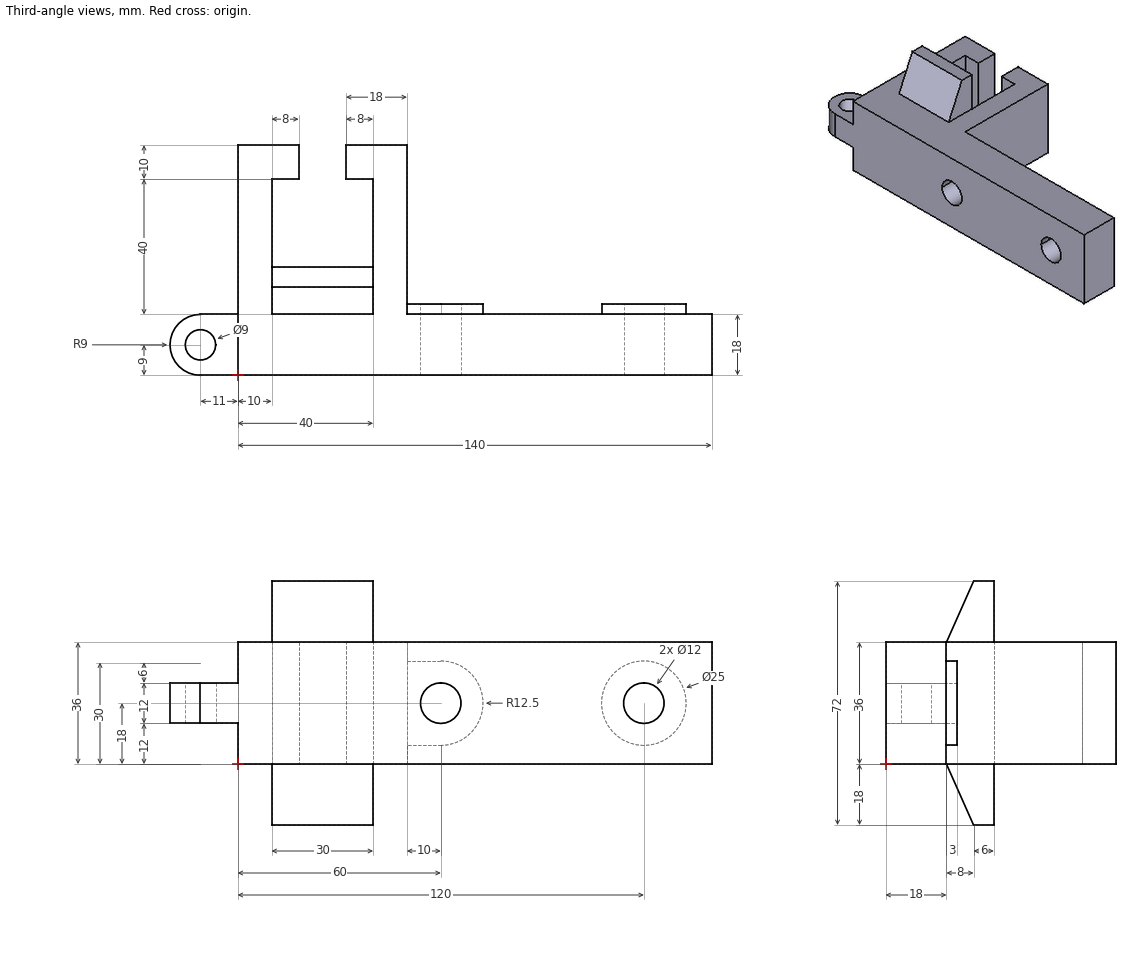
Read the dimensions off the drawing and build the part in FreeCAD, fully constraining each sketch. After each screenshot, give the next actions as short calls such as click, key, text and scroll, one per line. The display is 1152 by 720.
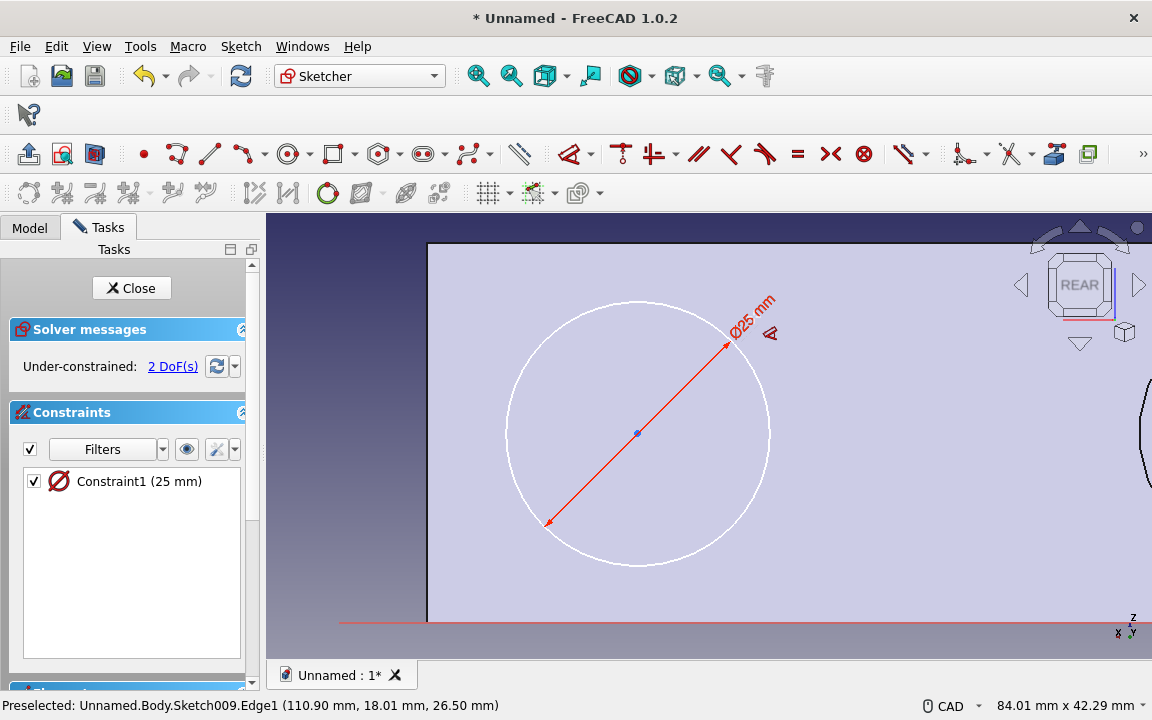
click(638, 434)
click(604, 528)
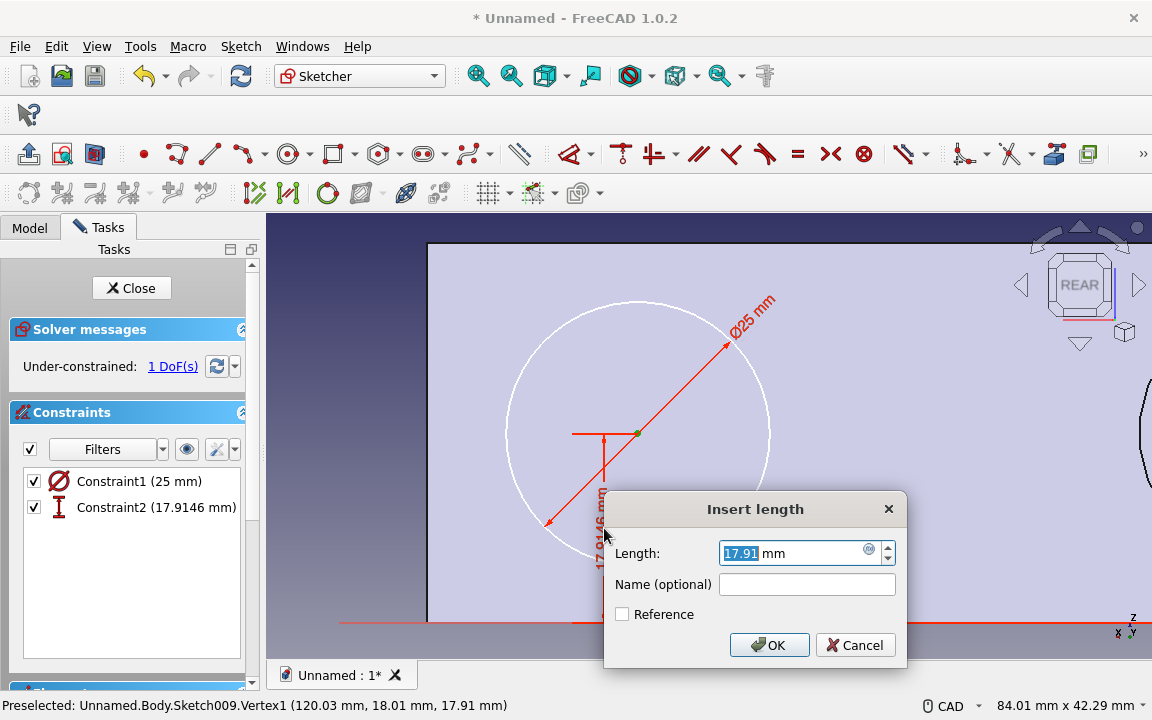
text(18)
key(Return)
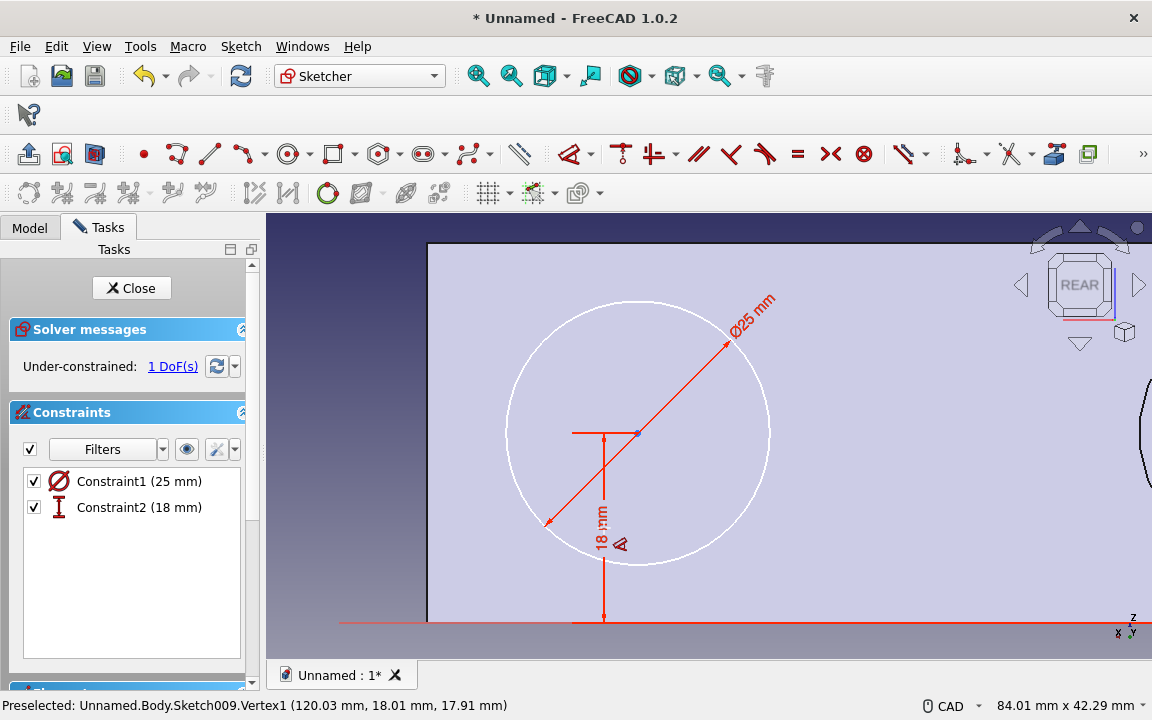
click(638, 433)
click(813, 399)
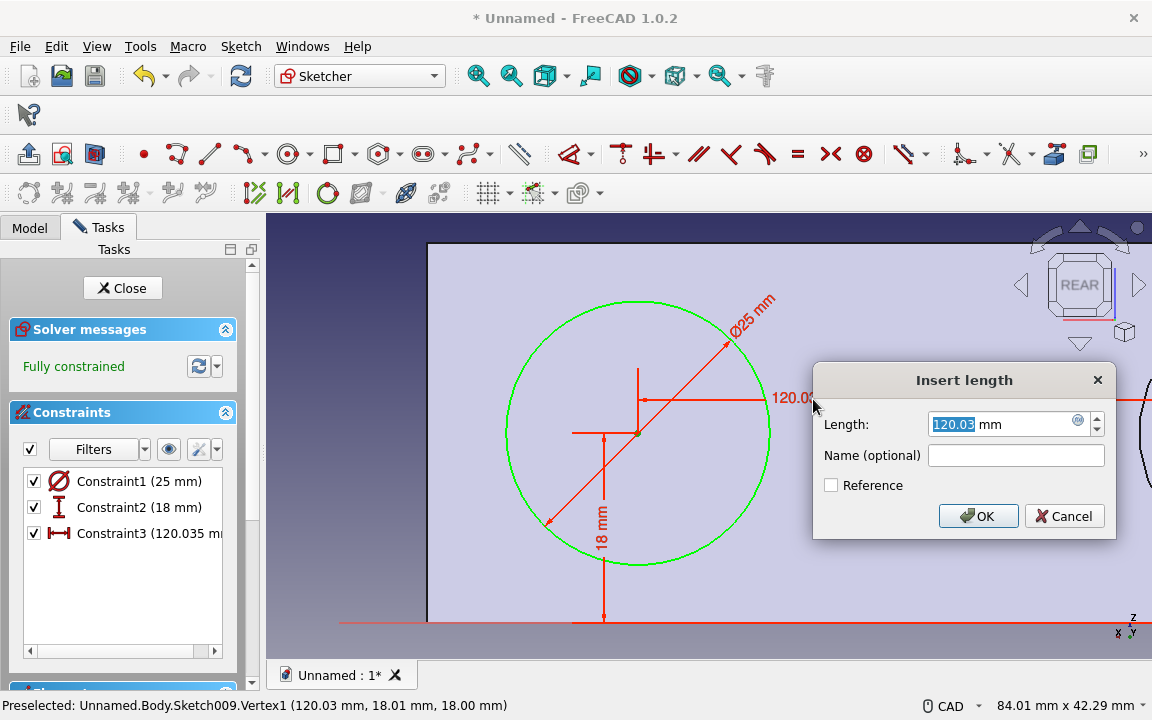
text(120)
key(Return)
key(Escape)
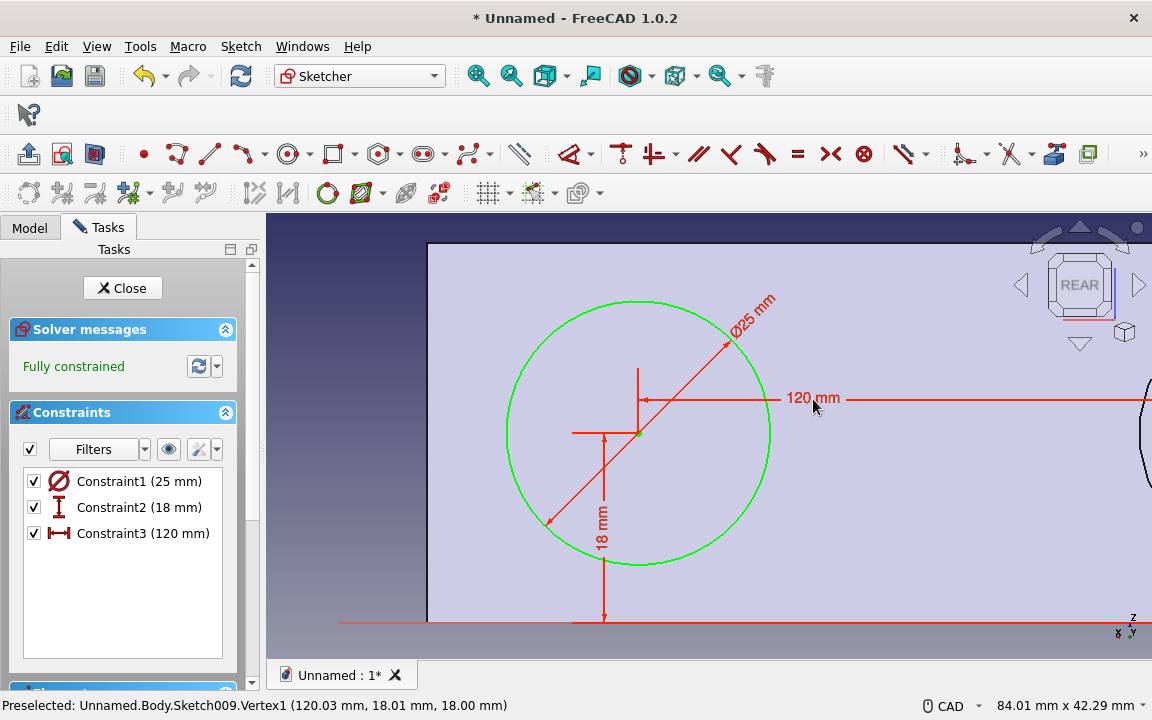
click(123, 288)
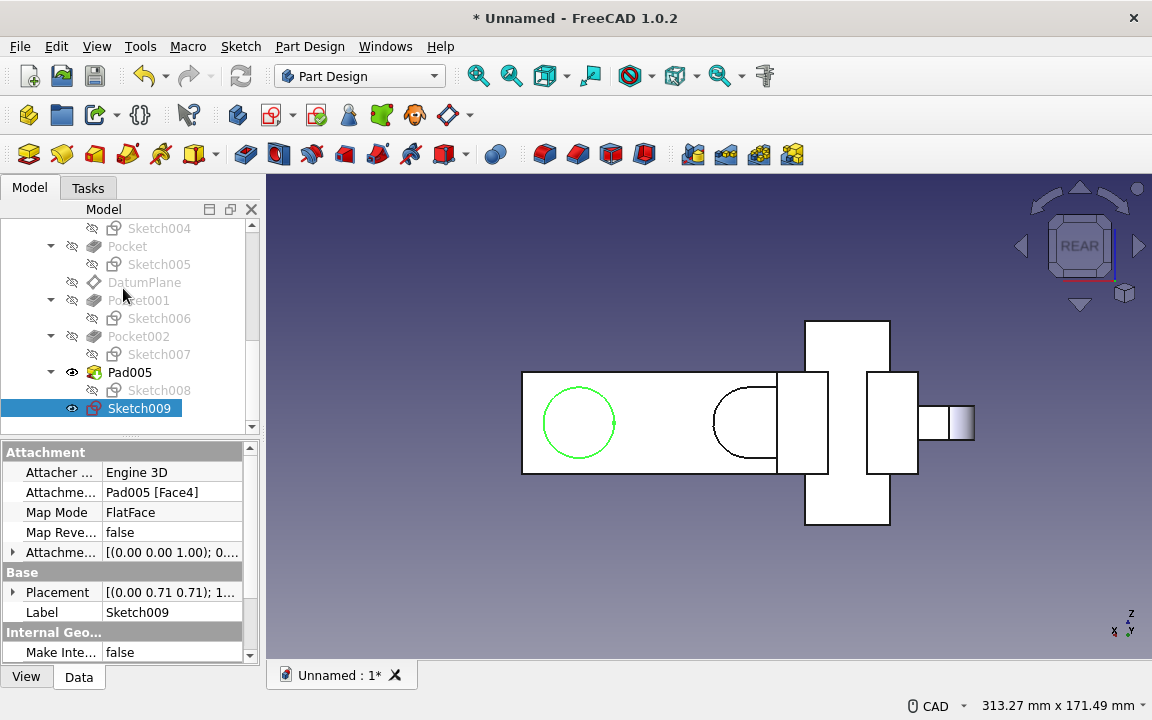
click(29, 154)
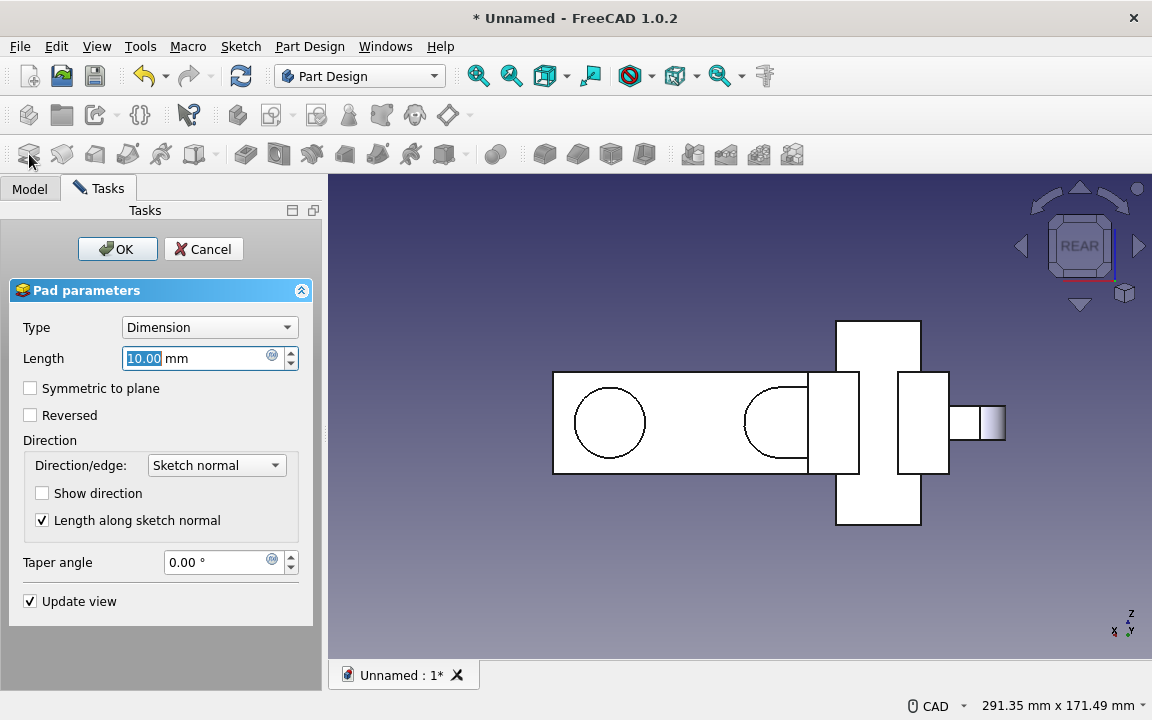
text(3)
key(Tab)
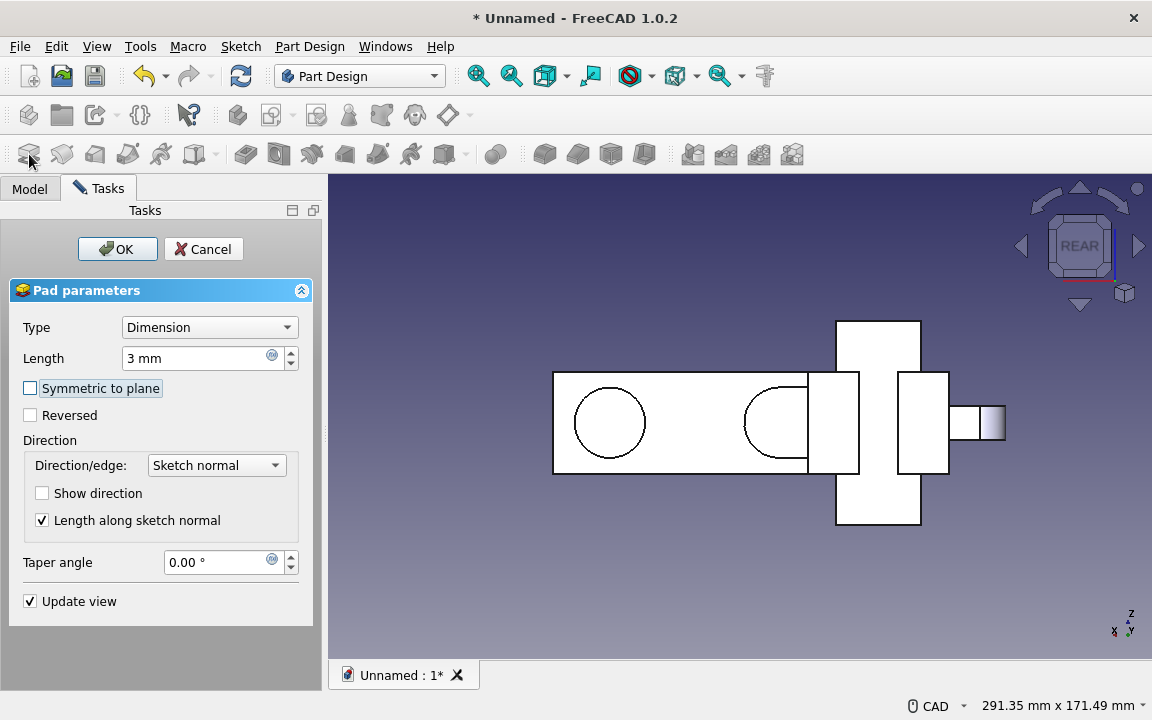
click(118, 249)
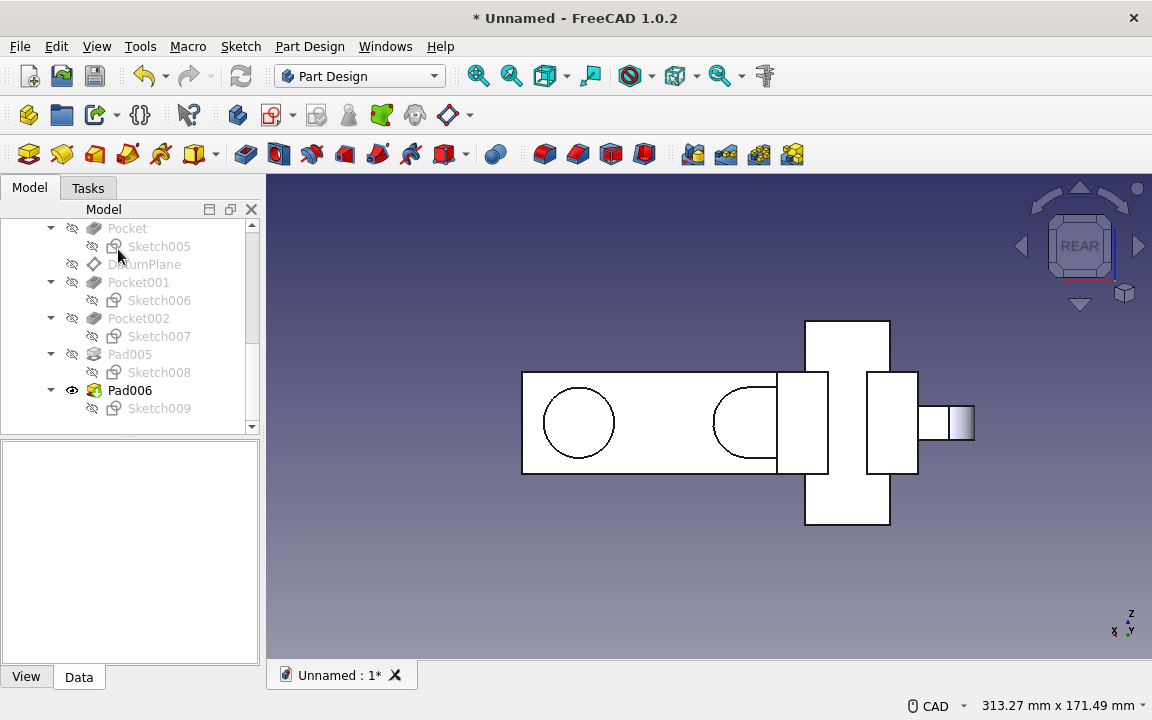
click(745, 422)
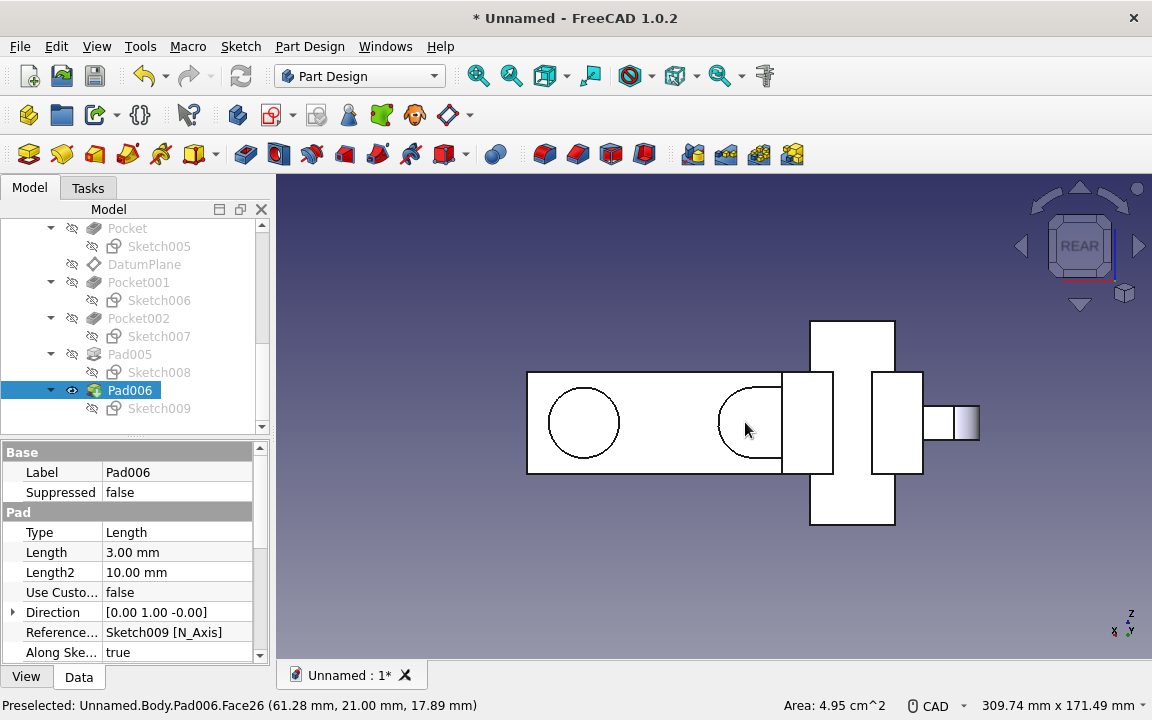
click(270, 116)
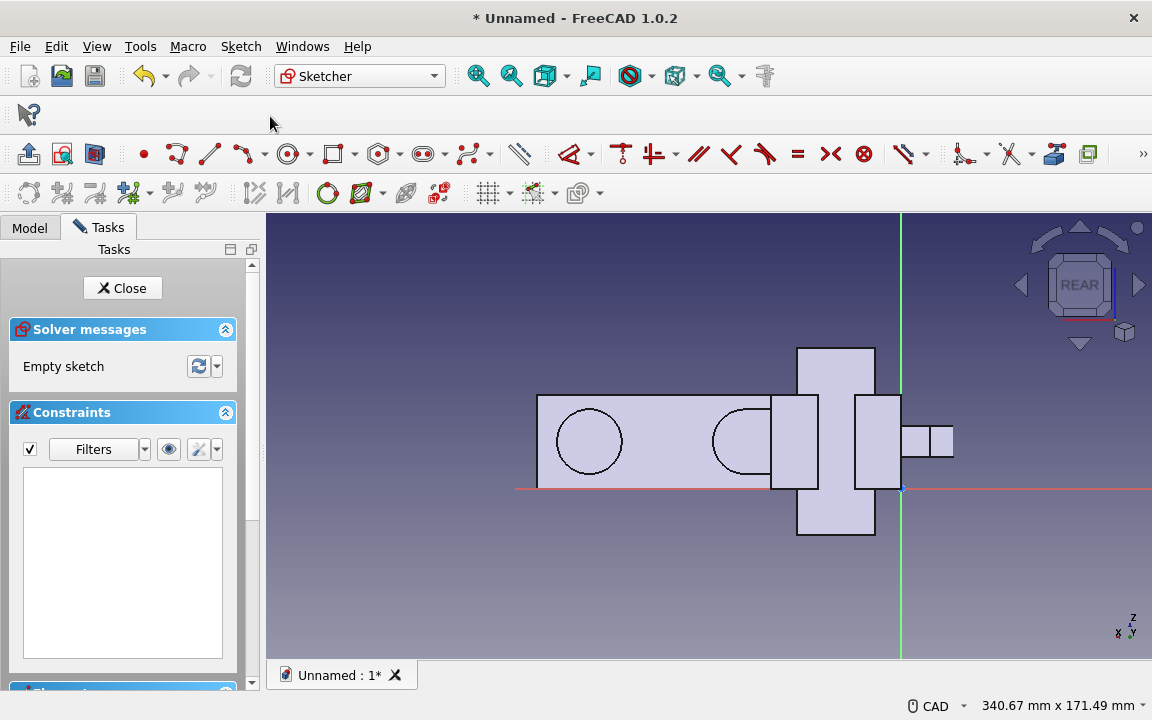
scroll(935, 501, up, 2)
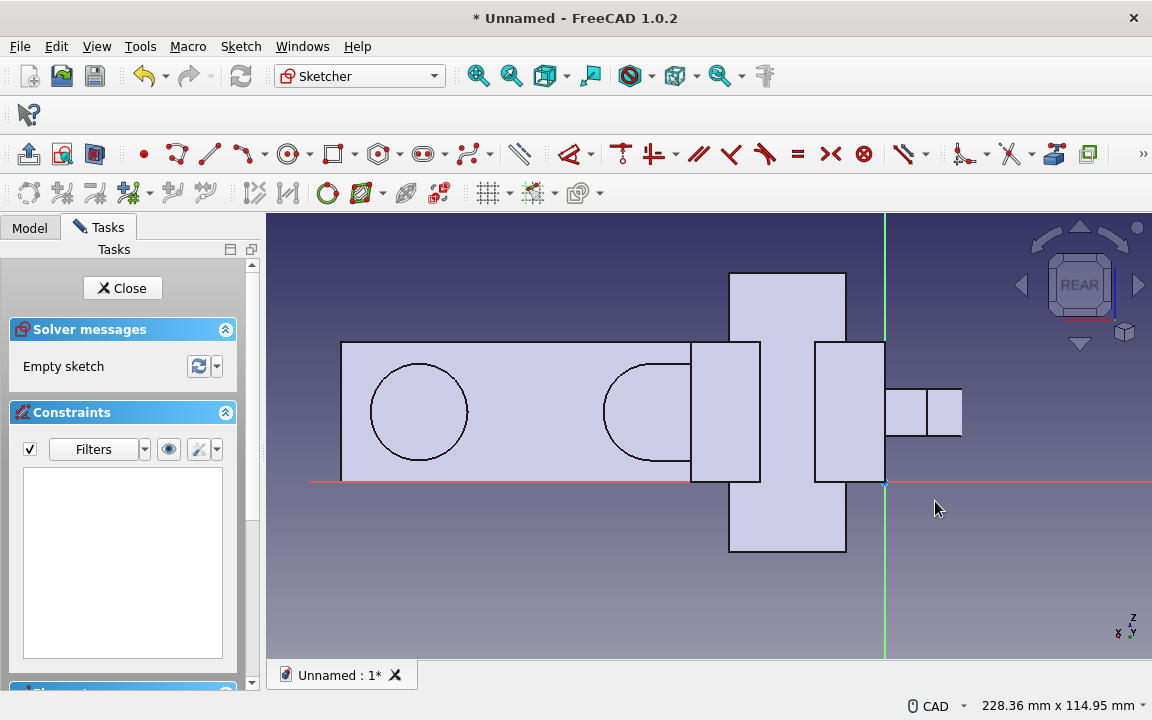
key(g)
key(c)